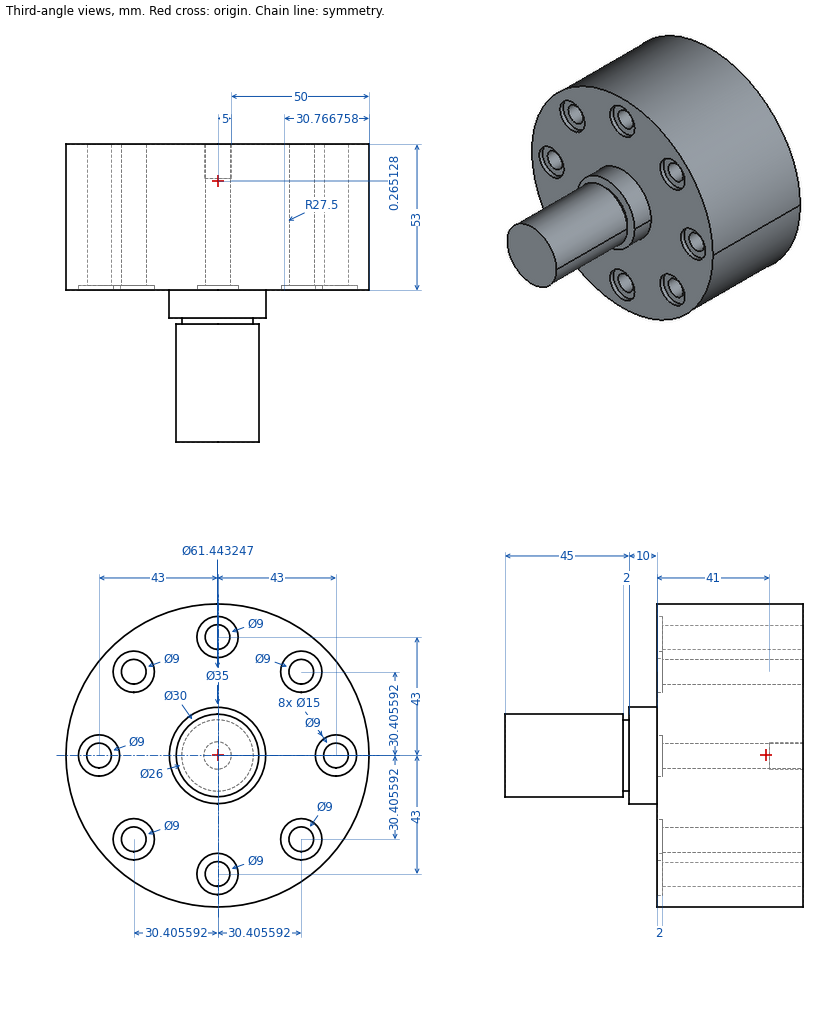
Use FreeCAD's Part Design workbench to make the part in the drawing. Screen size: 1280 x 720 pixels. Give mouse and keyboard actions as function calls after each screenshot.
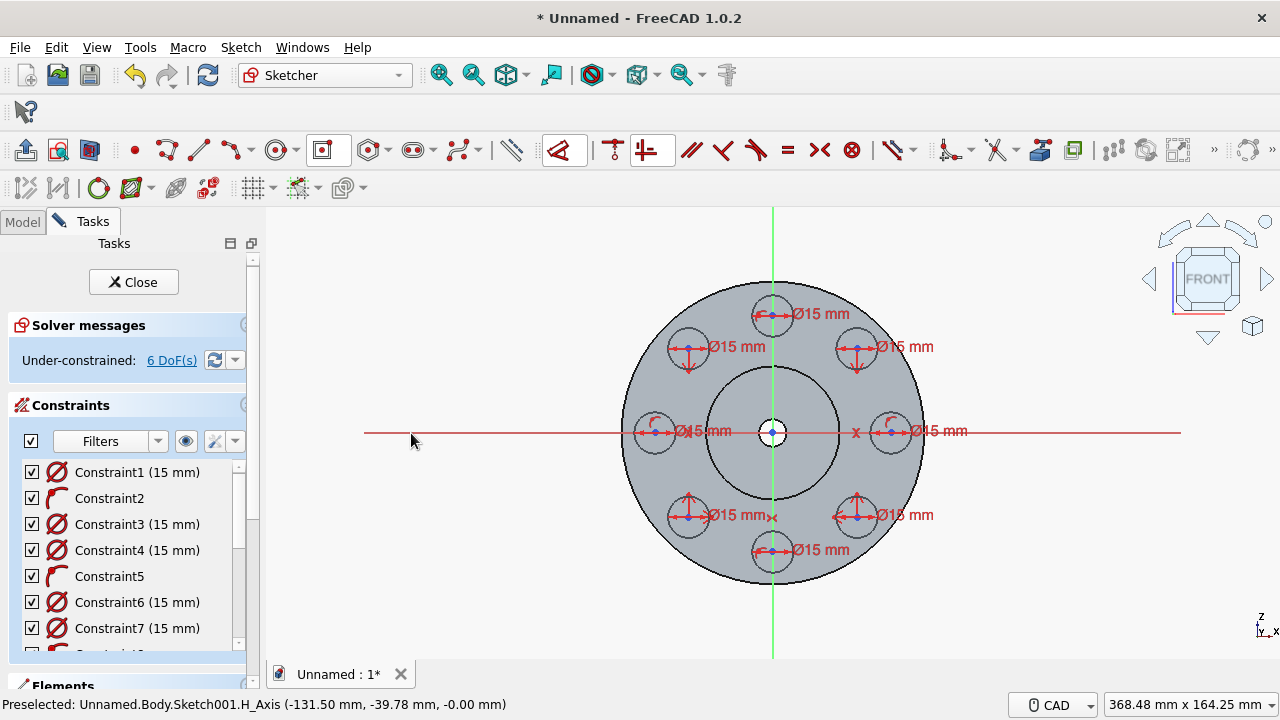
click(891, 433)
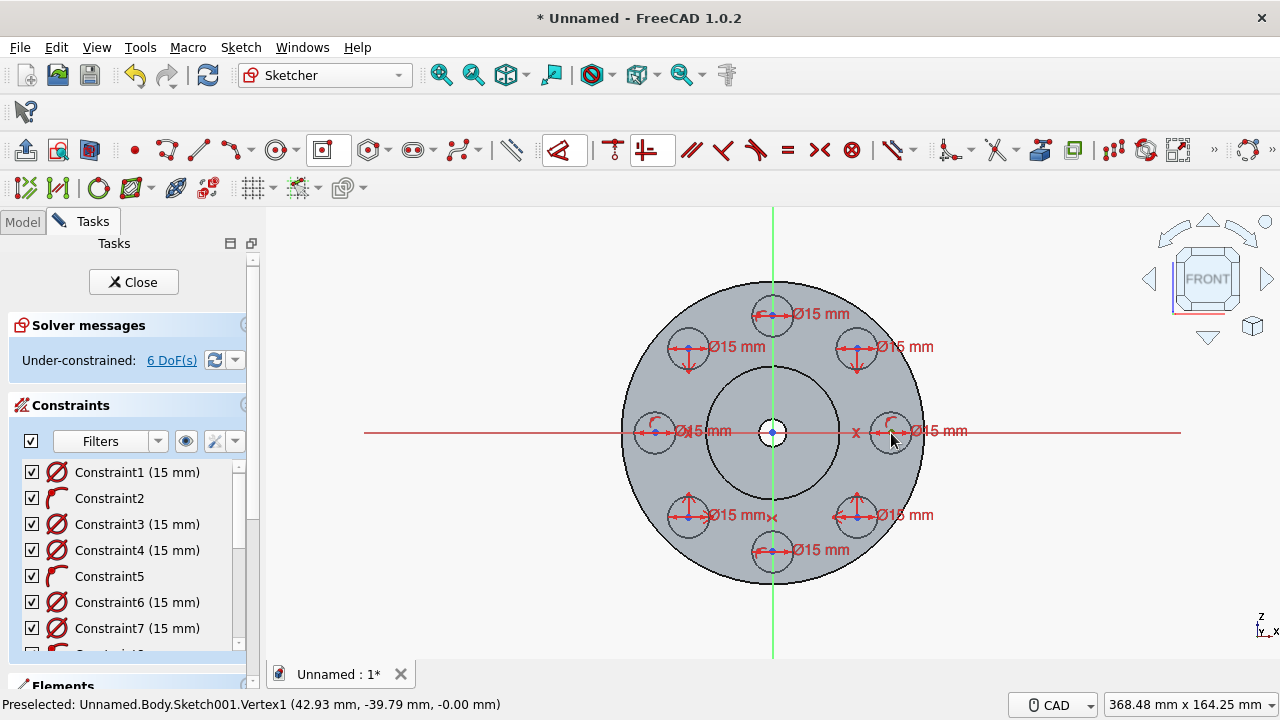
click(582, 150)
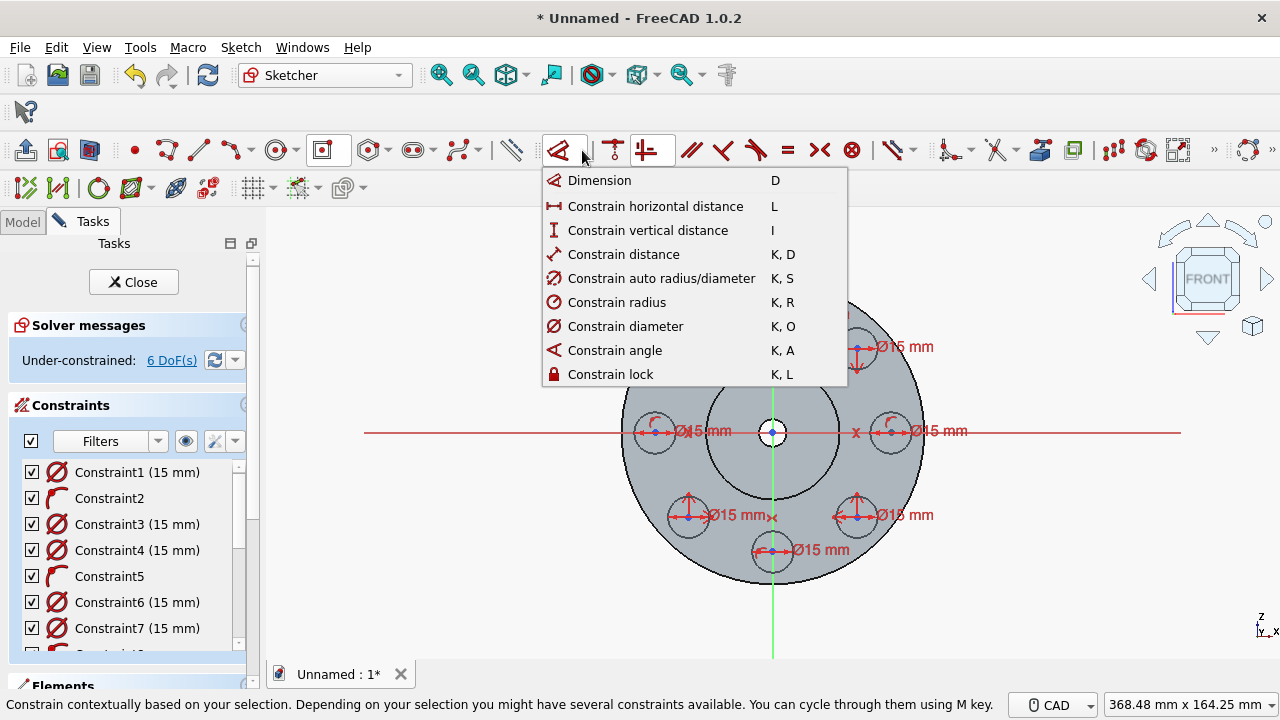
click(695, 206)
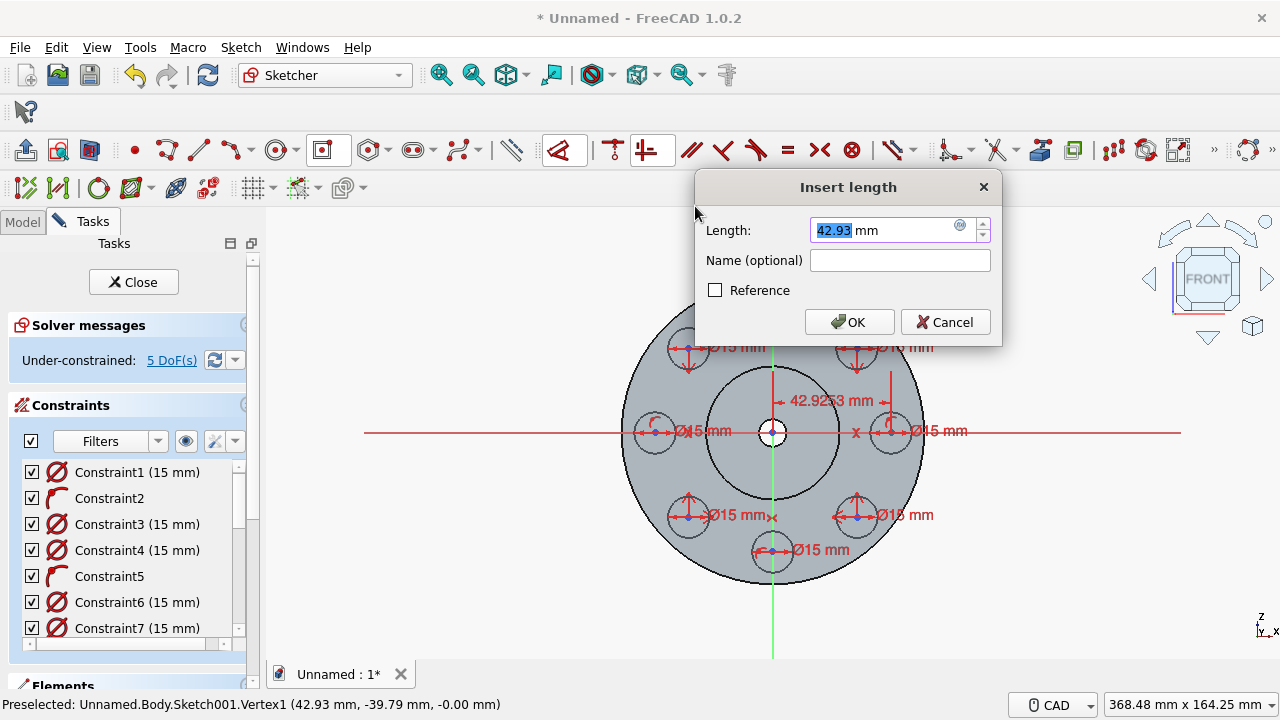
text(43)
key(Return)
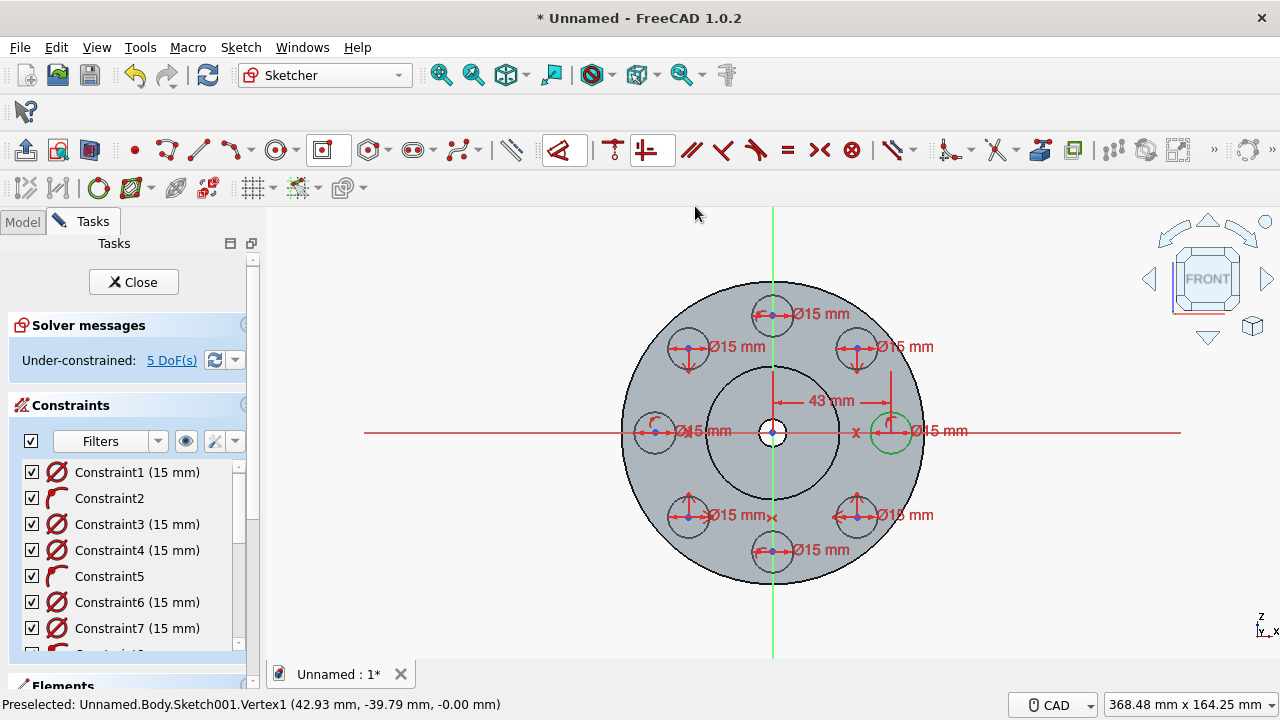
click(773, 552)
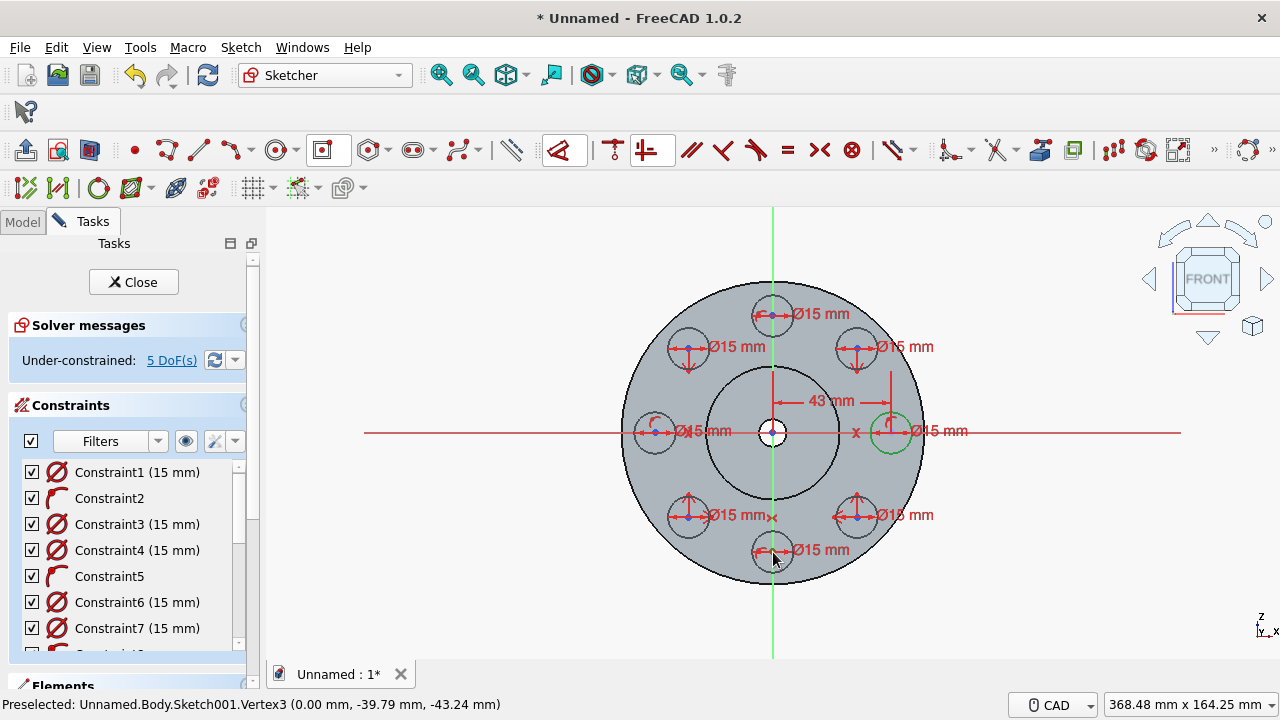
click(582, 150)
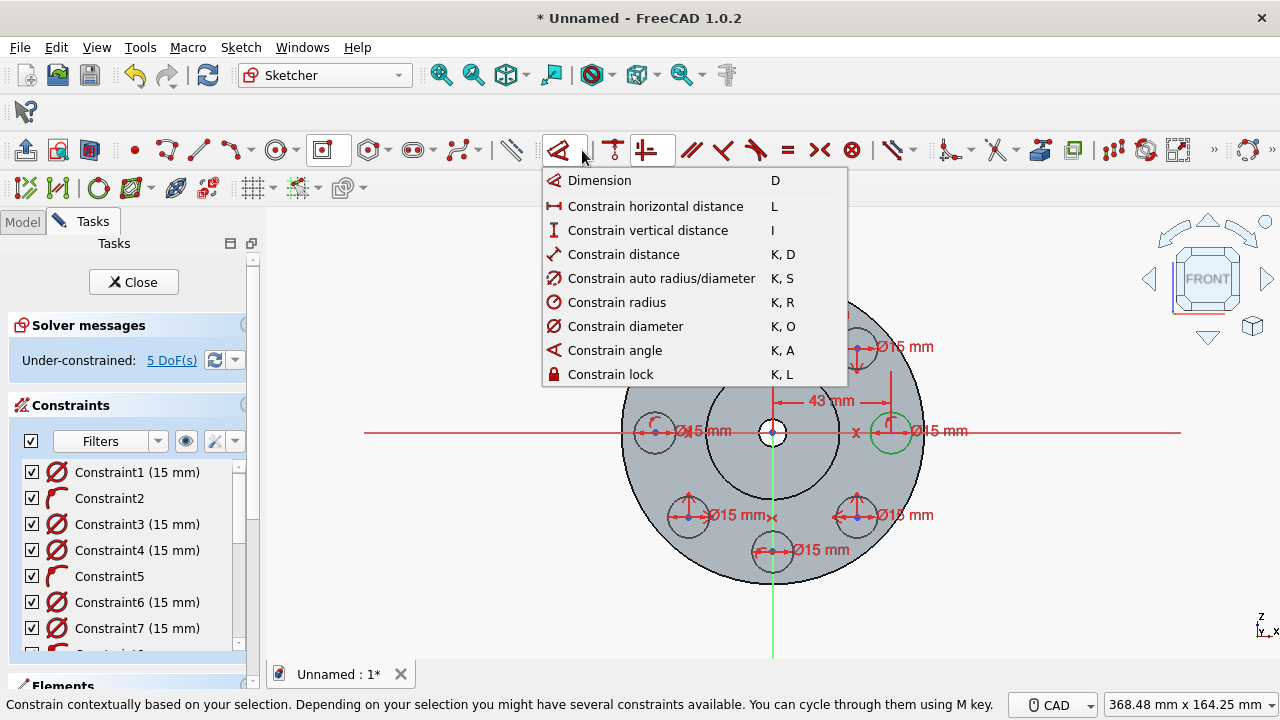
click(695, 230)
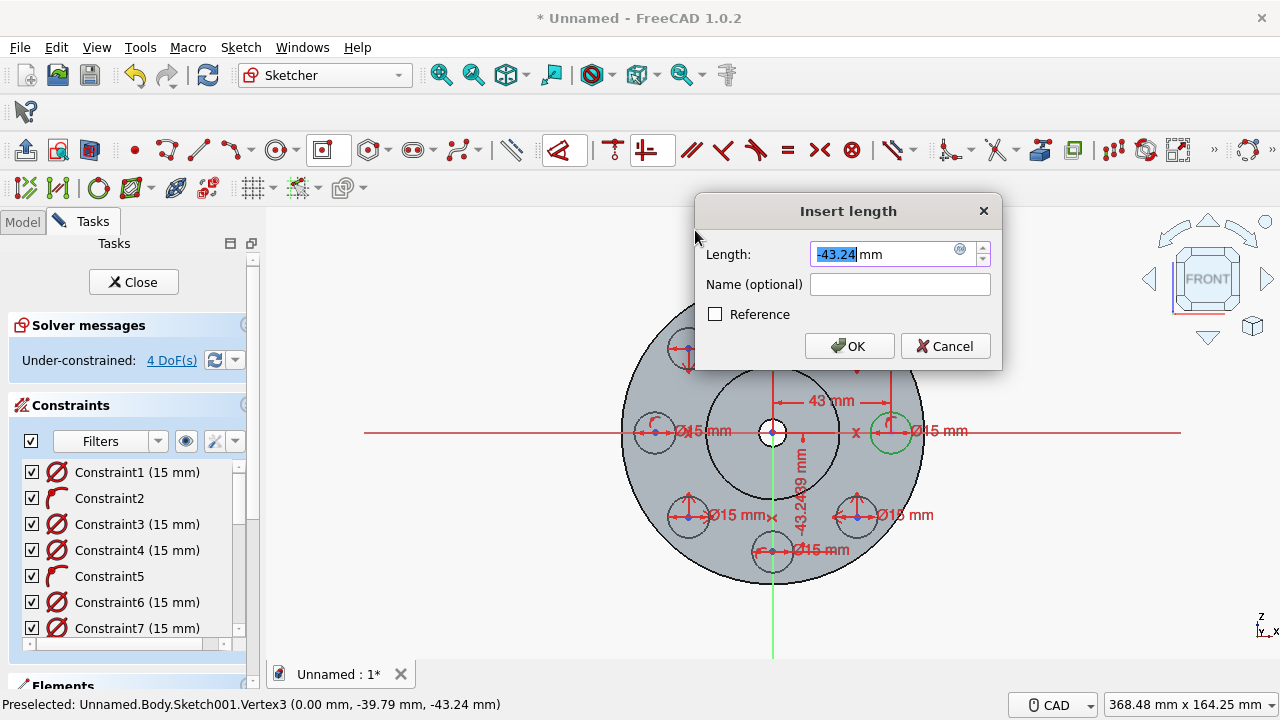
text(-43)
key(Return)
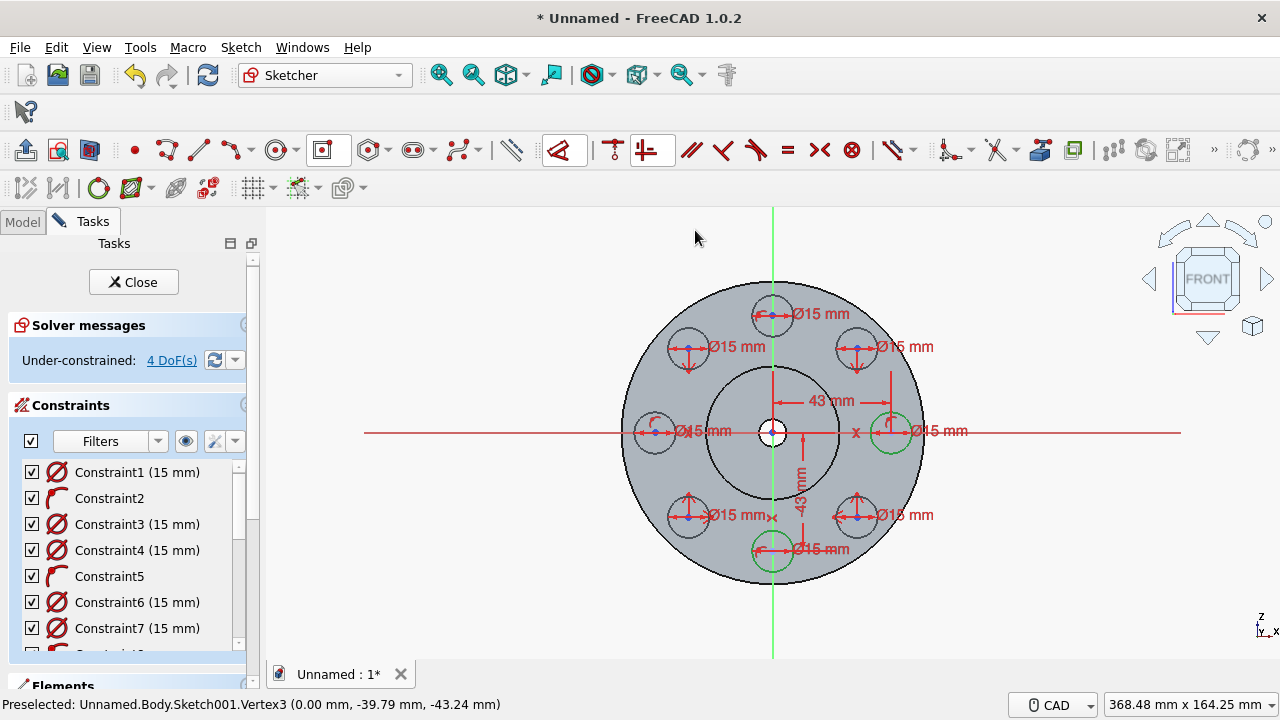
click(655, 433)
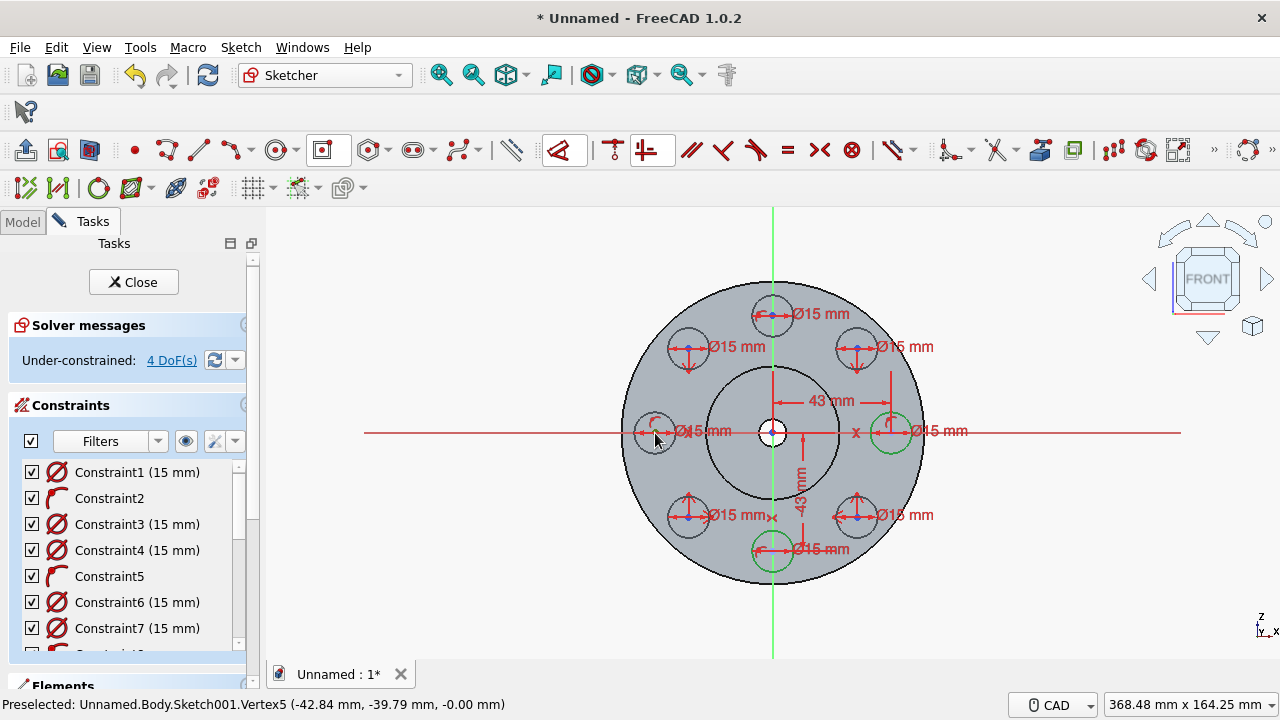
key(l)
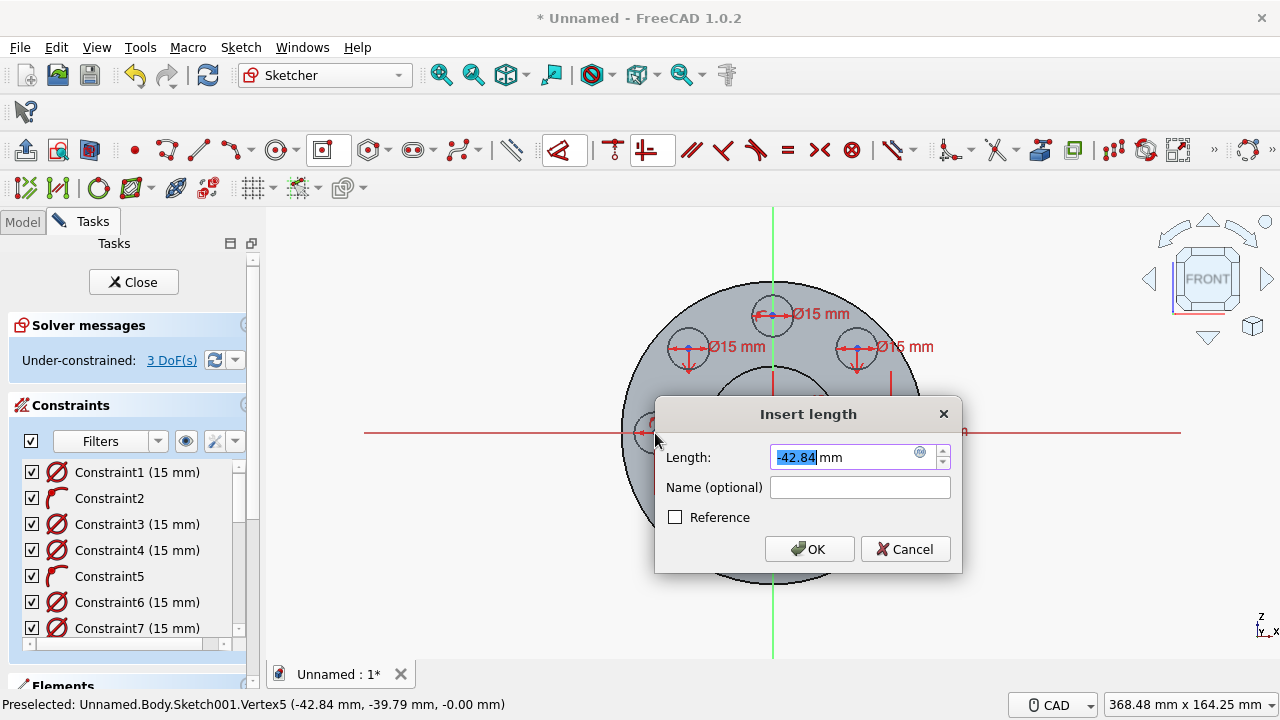
text(-43)
key(Return)